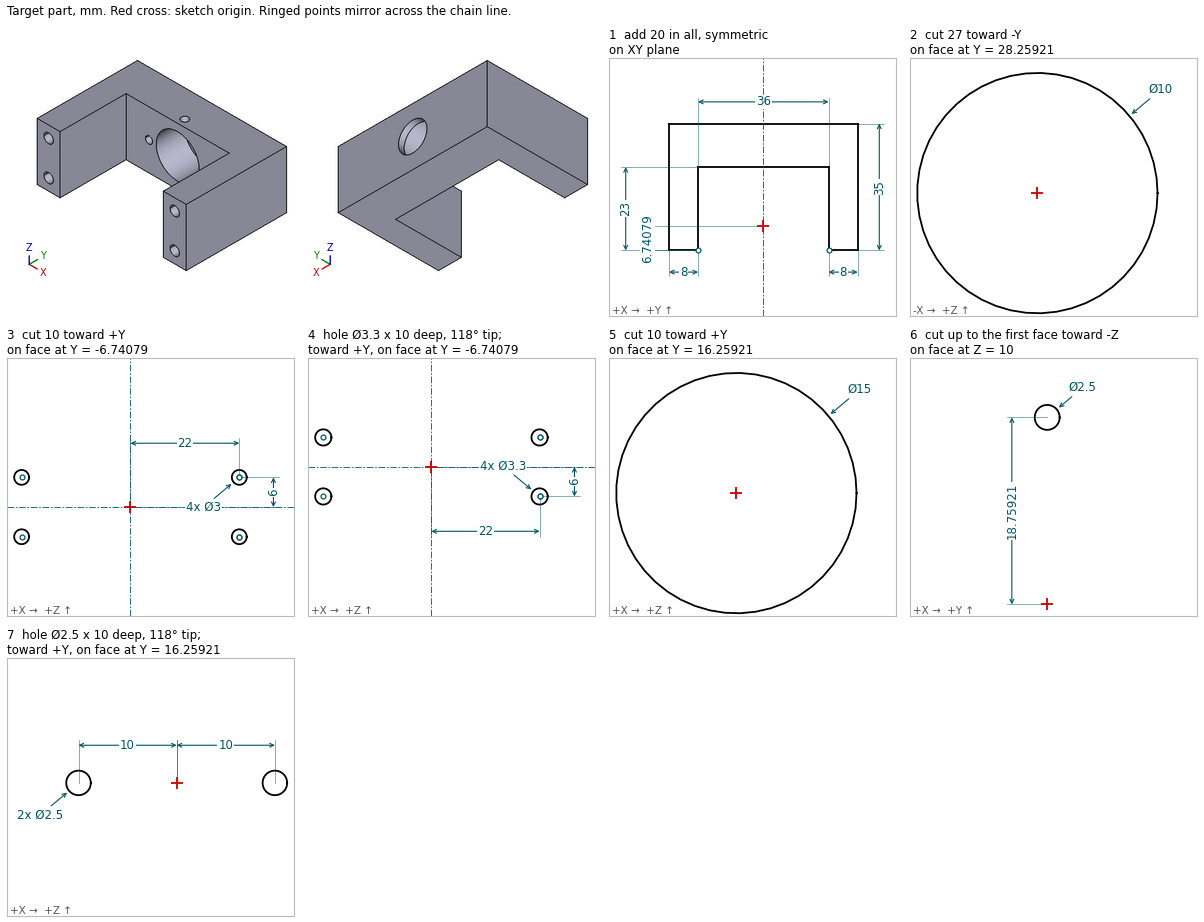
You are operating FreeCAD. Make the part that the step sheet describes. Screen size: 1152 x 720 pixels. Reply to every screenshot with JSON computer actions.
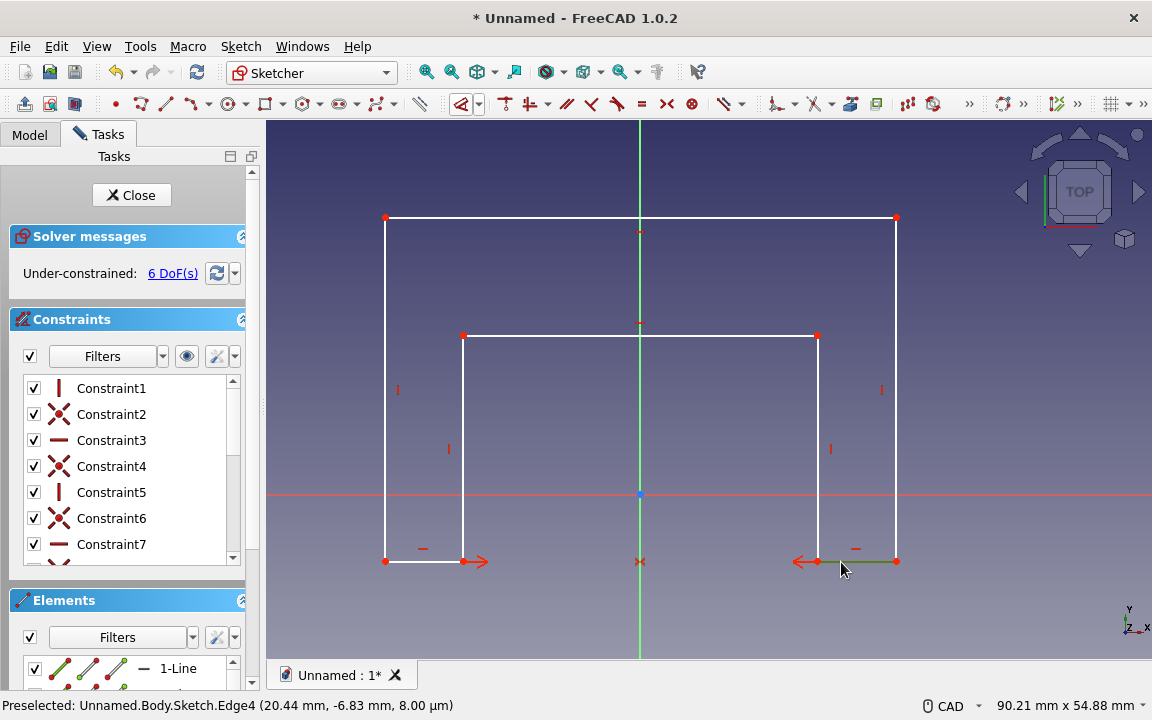
{"action": "key", "text": "l"}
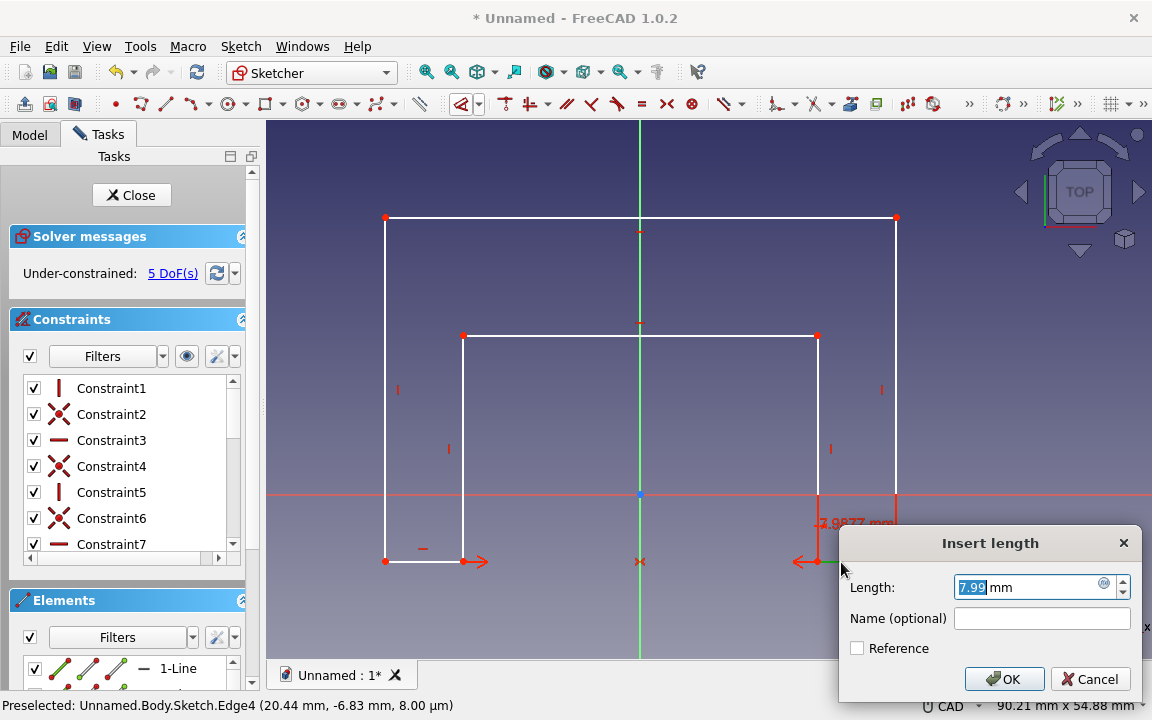
{"action": "type", "text": "8"}
{"action": "key", "text": "Return"}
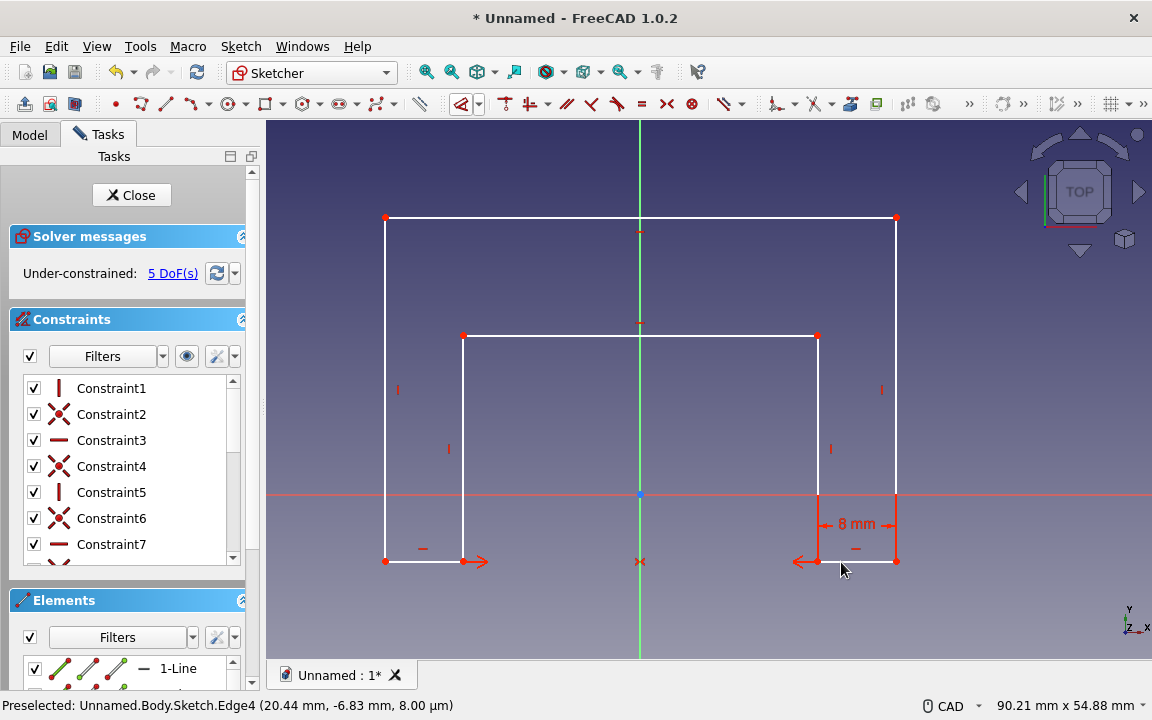
{"action": "left_click", "coordinate": [408, 562]}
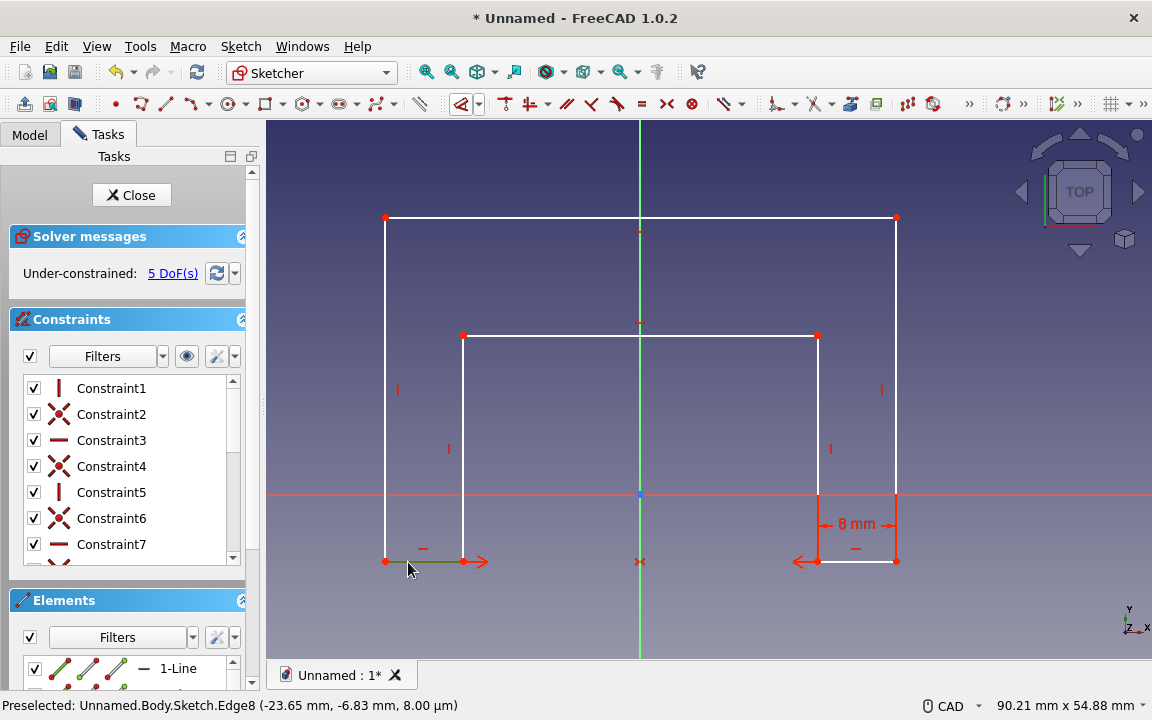
{"action": "key", "text": "l"}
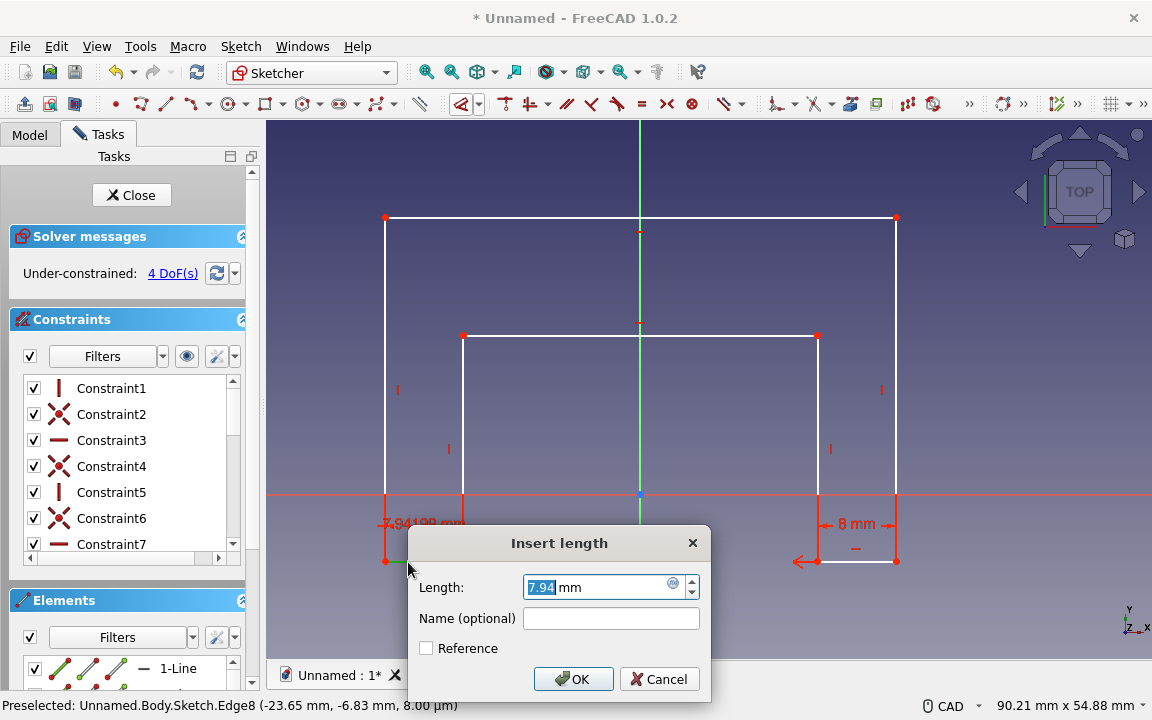
{"action": "type", "text": "8"}
{"action": "key", "text": "Return"}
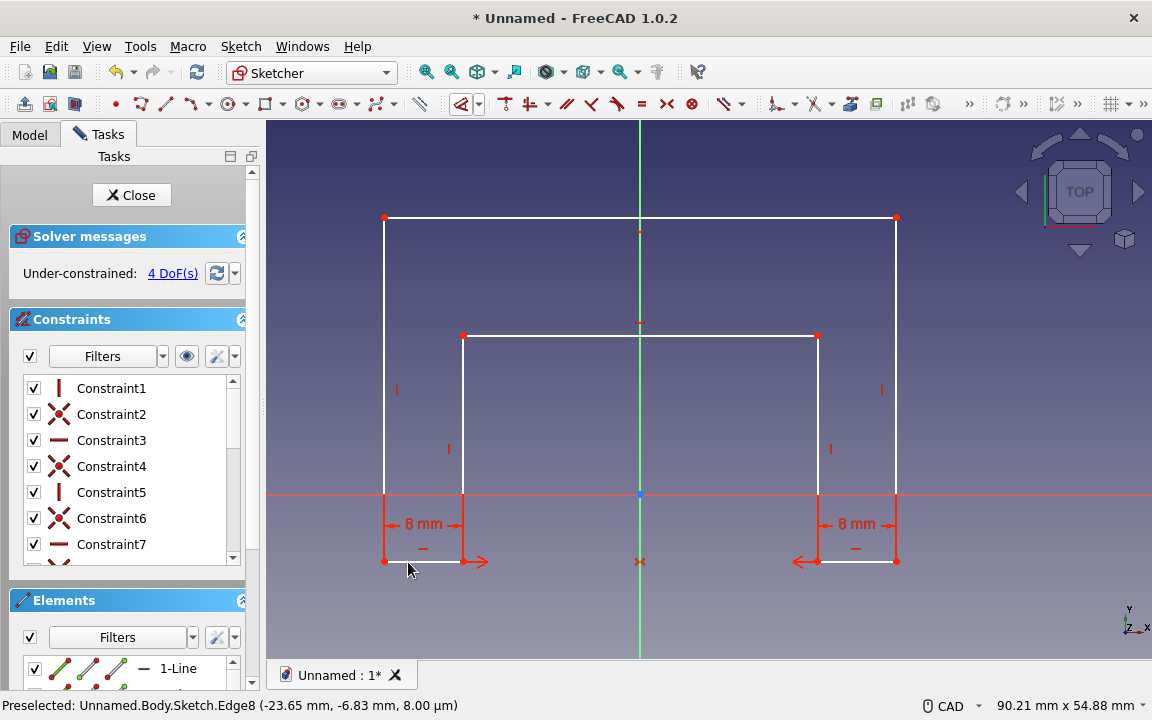
{"action": "left_click", "coordinate": [463, 494]}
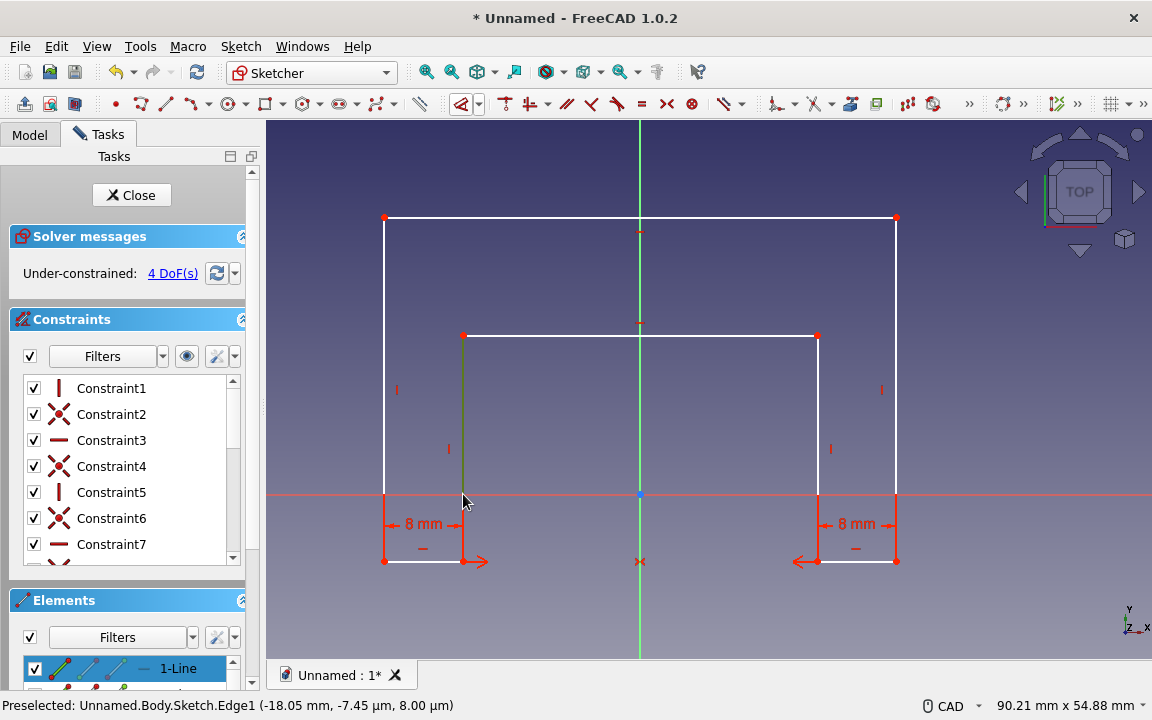
{"action": "left_click", "coordinate": [478, 104]}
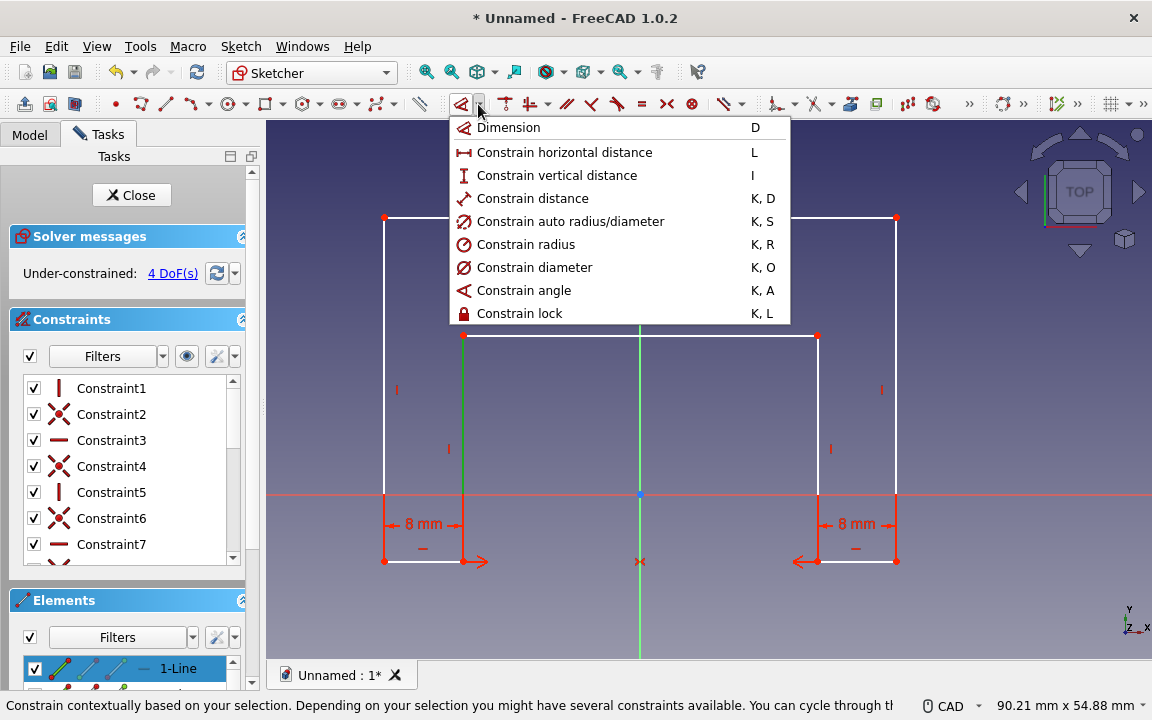
{"action": "left_click", "coordinate": [620, 176]}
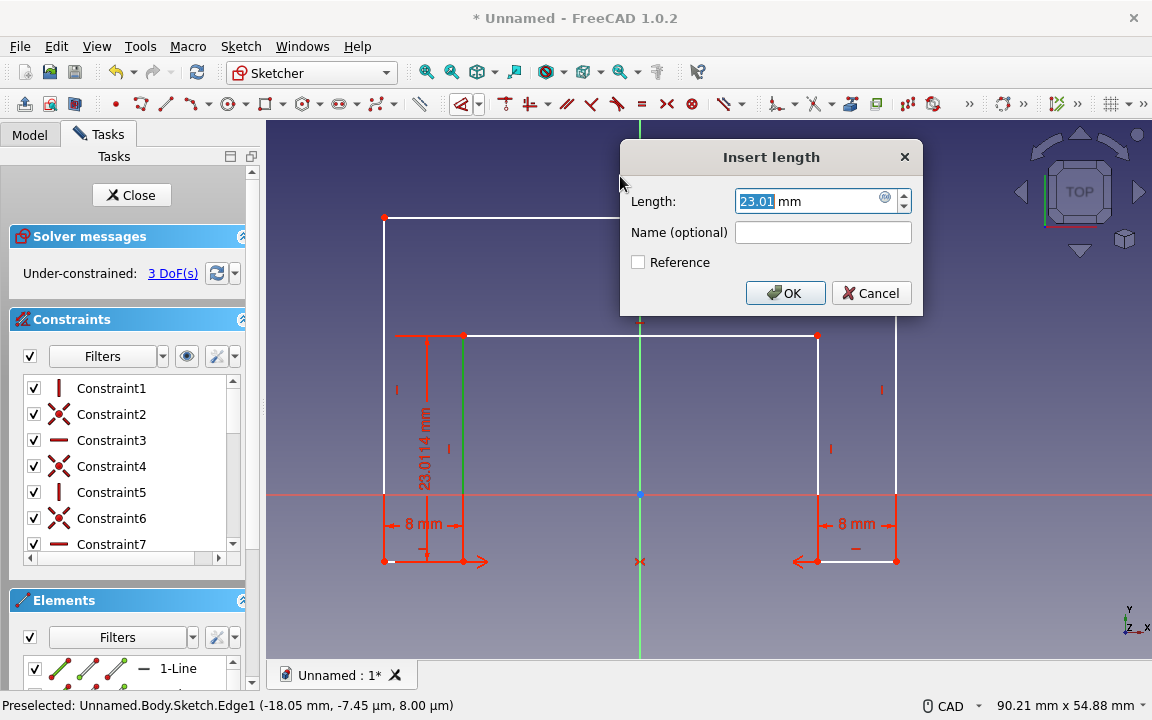
{"action": "type", "text": "23"}
{"action": "key", "text": "Return"}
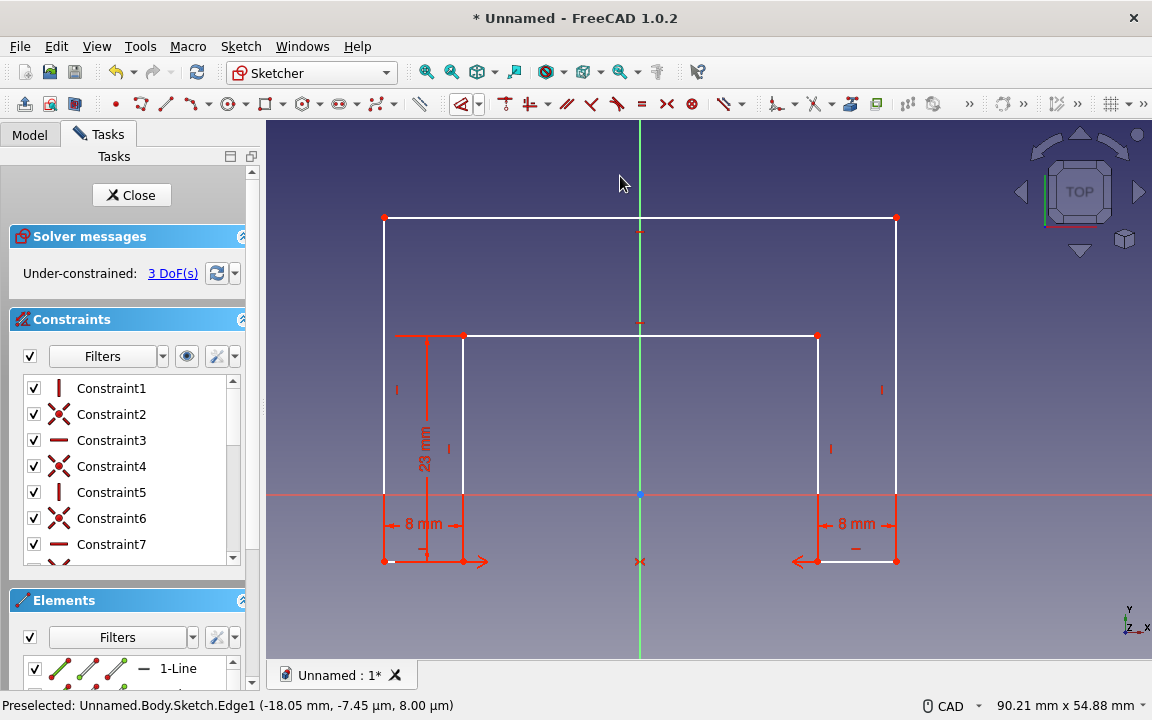
{"action": "left_click", "coordinate": [569, 336]}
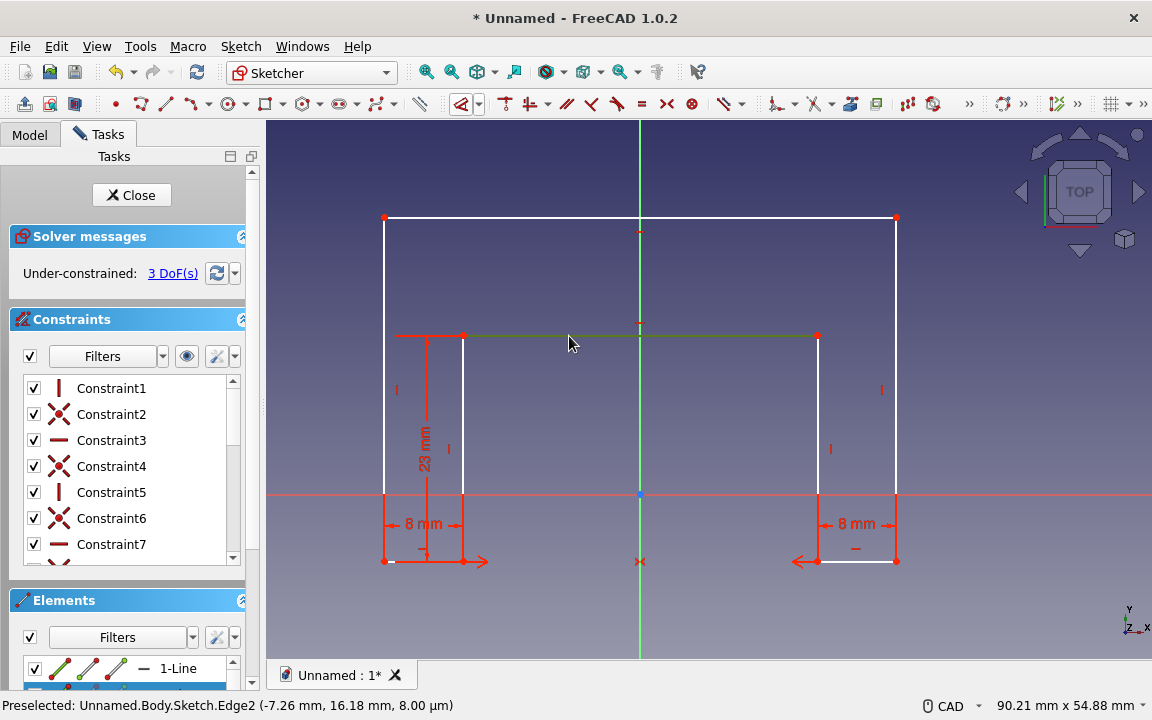
{"action": "key", "text": "l"}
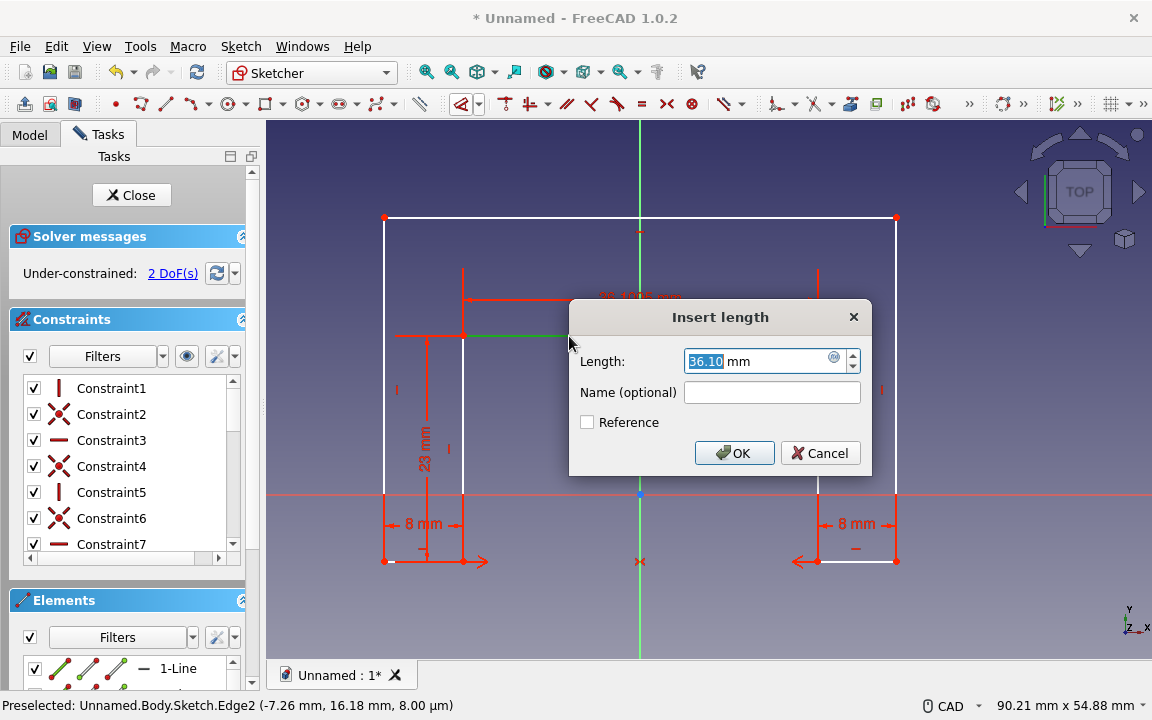
{"action": "type", "text": "36"}
{"action": "key", "text": "Return"}